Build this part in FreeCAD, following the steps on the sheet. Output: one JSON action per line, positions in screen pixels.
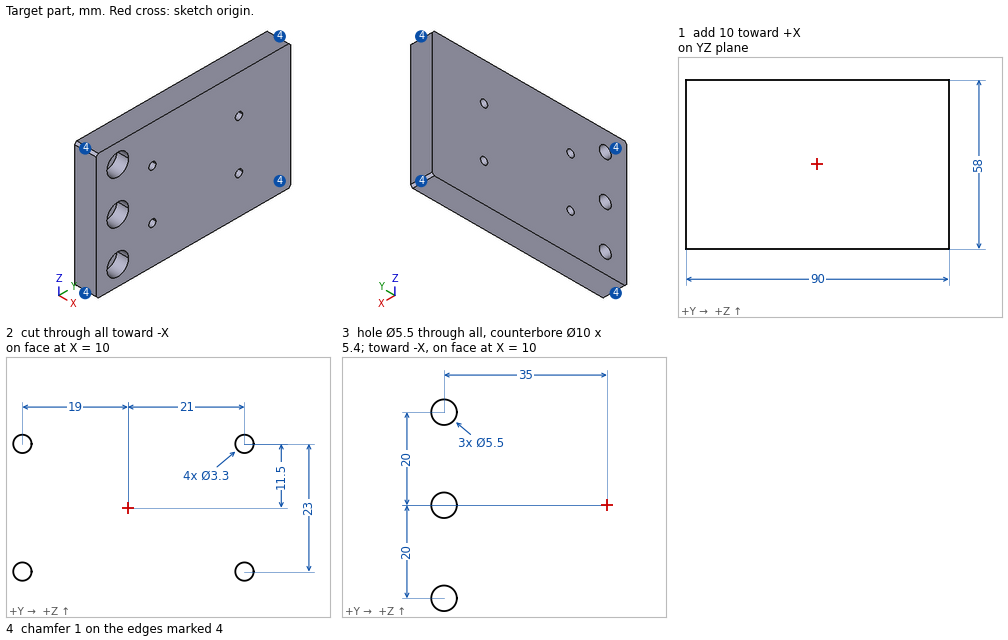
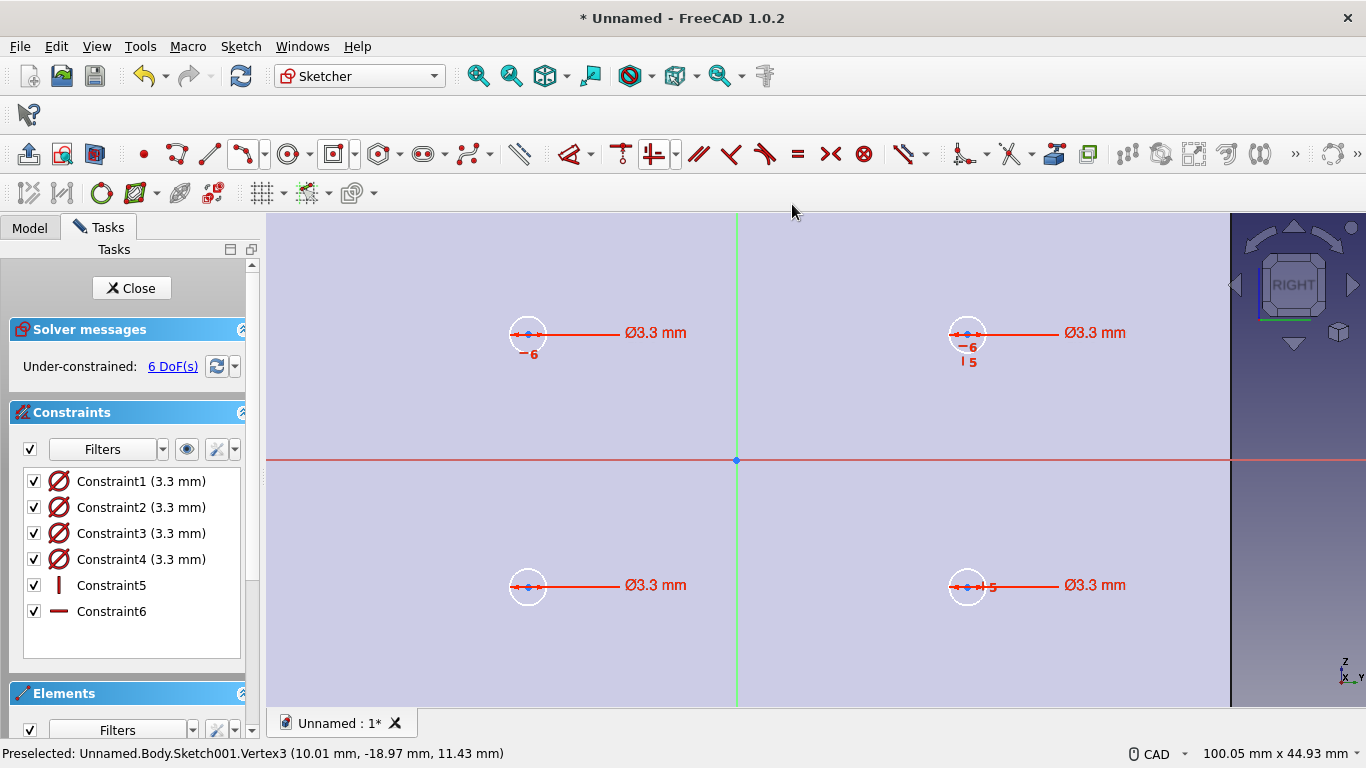
{"action": "left_click", "coordinate": [528, 335]}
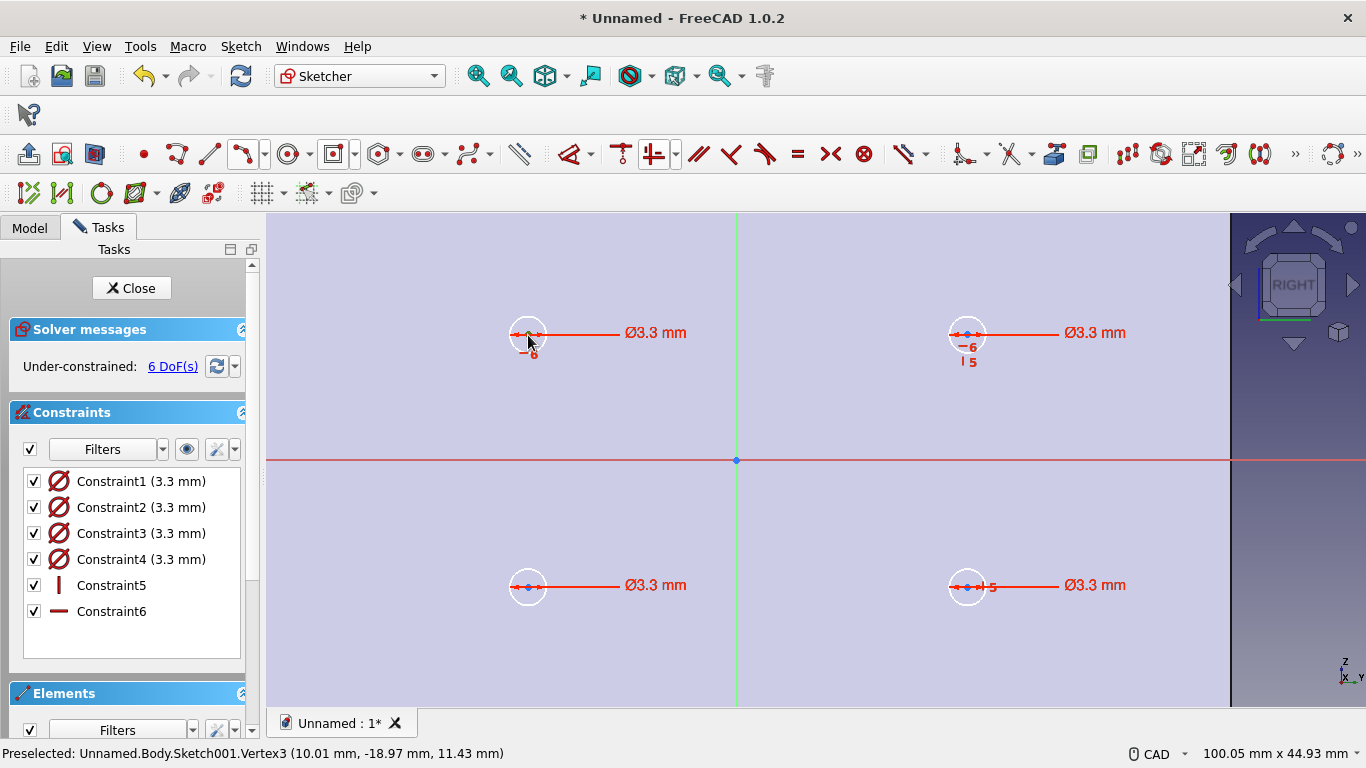
{"action": "left_click", "coordinate": [528, 587]}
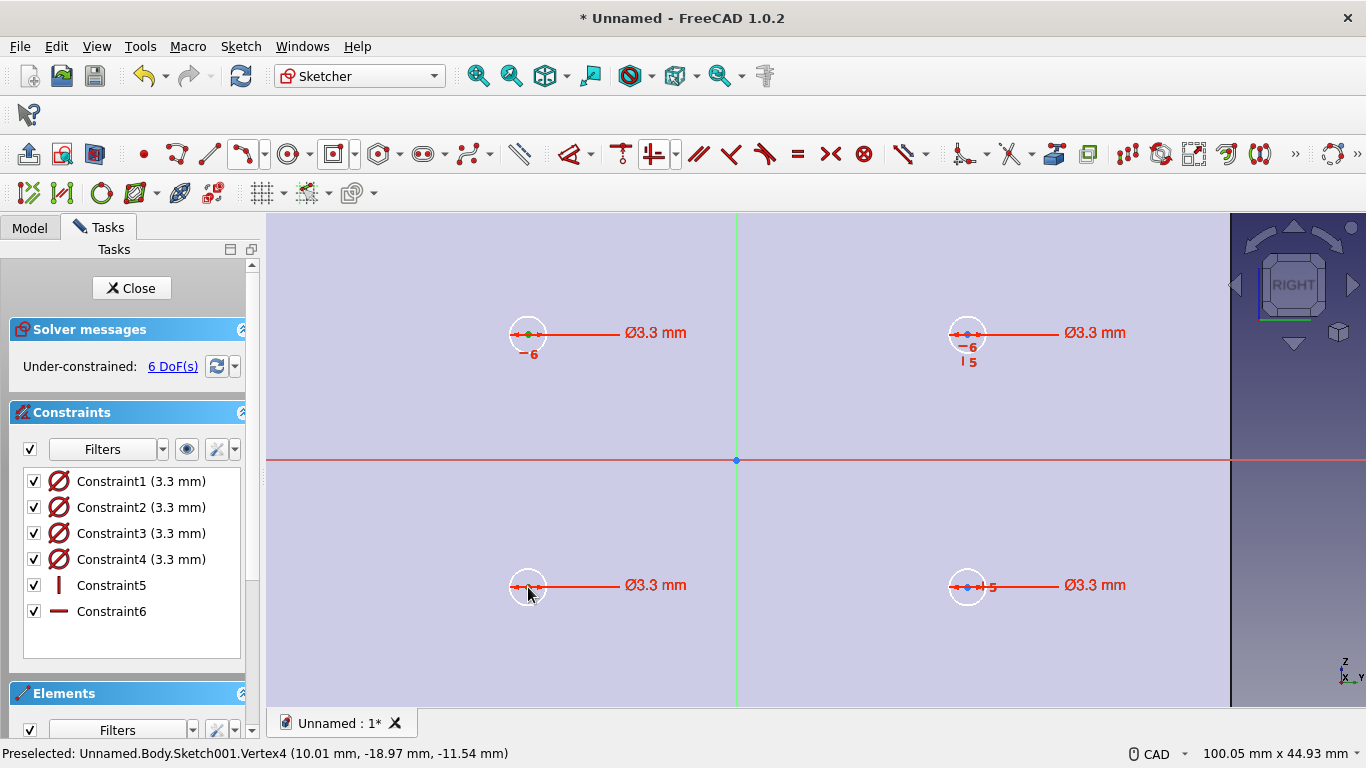
{"action": "left_click", "coordinate": [676, 154]}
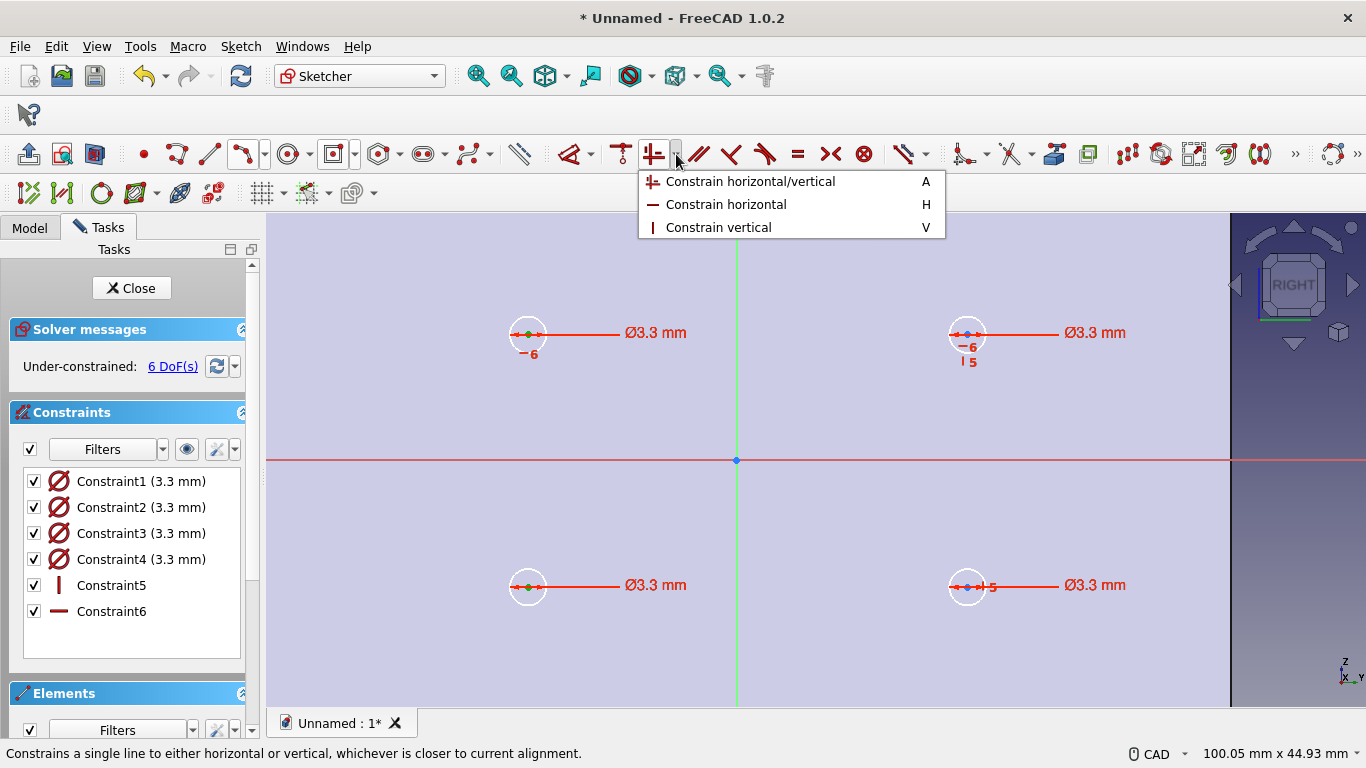
{"action": "left_click", "coordinate": [792, 228]}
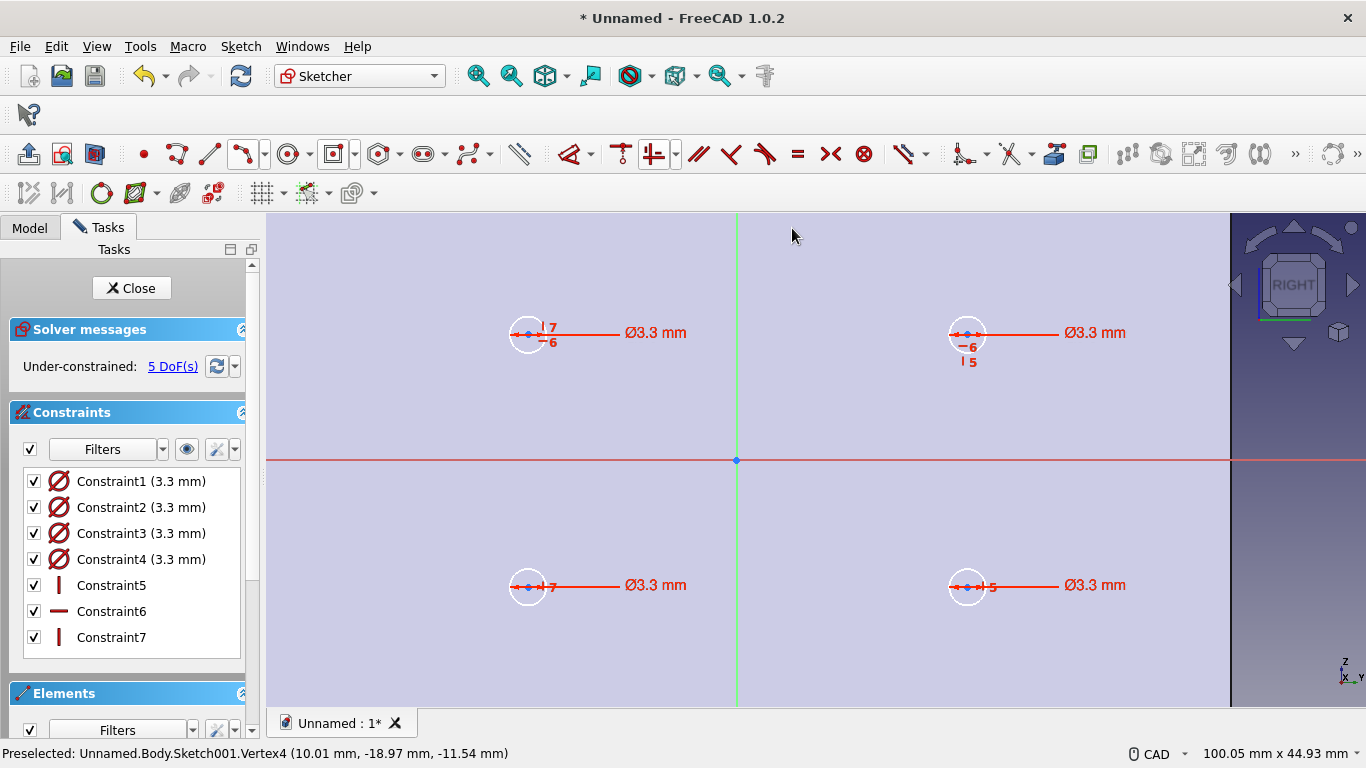
{"action": "left_click", "coordinate": [968, 587]}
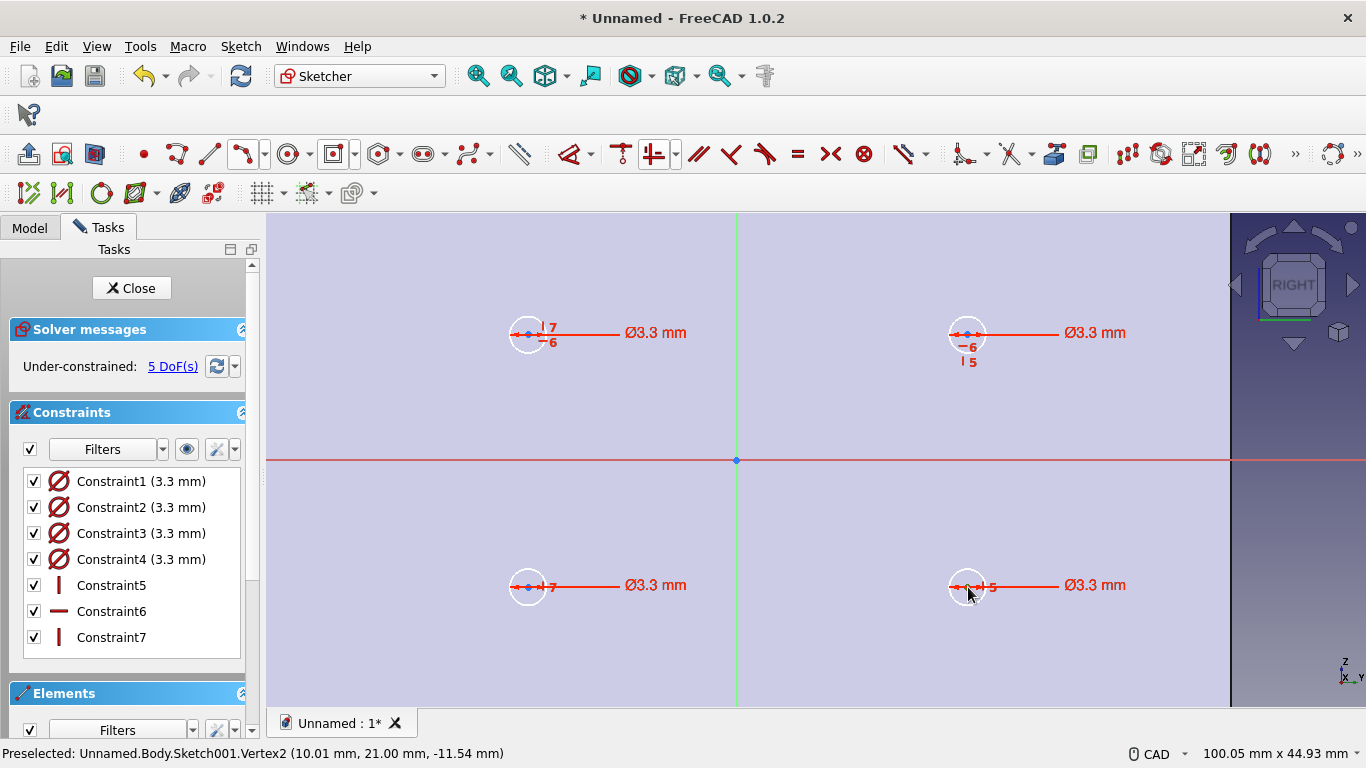
{"action": "left_click", "coordinate": [528, 587]}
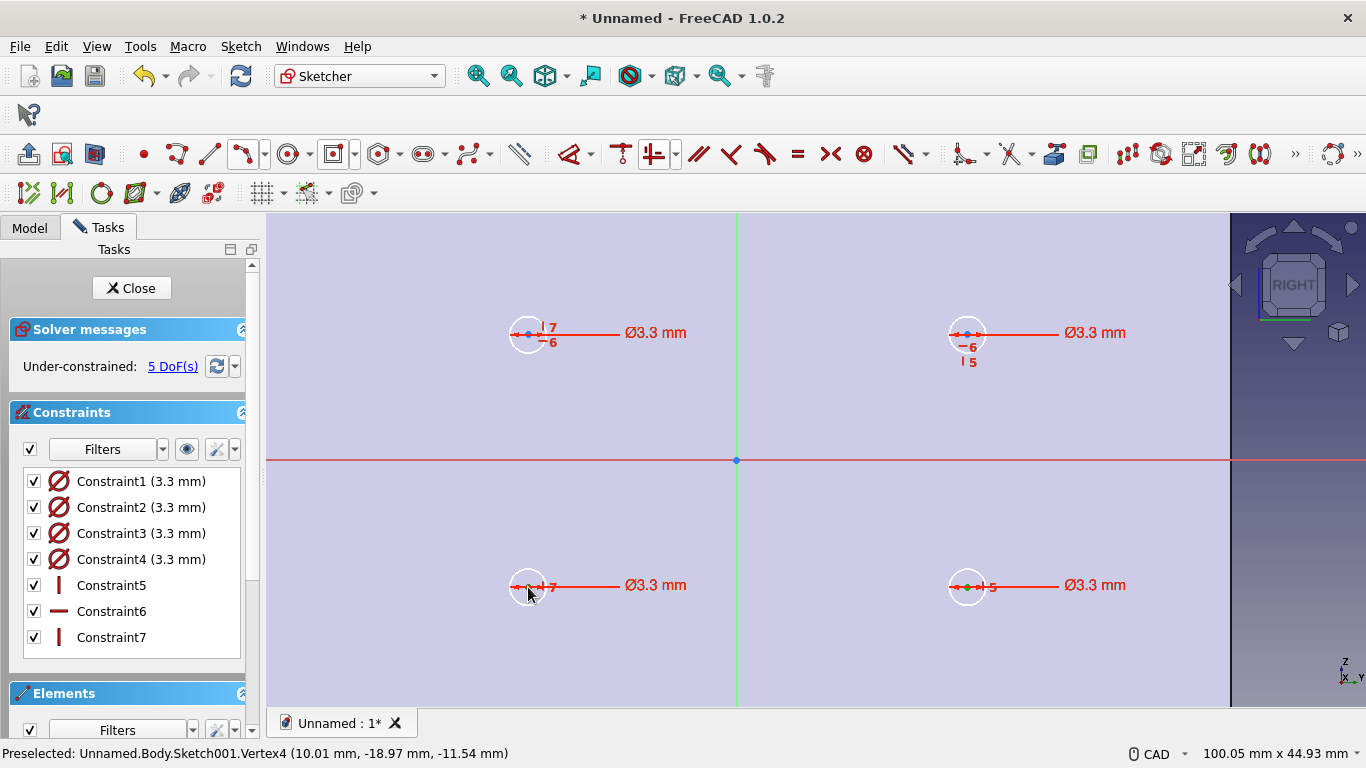
{"action": "left_click", "coordinate": [676, 154]}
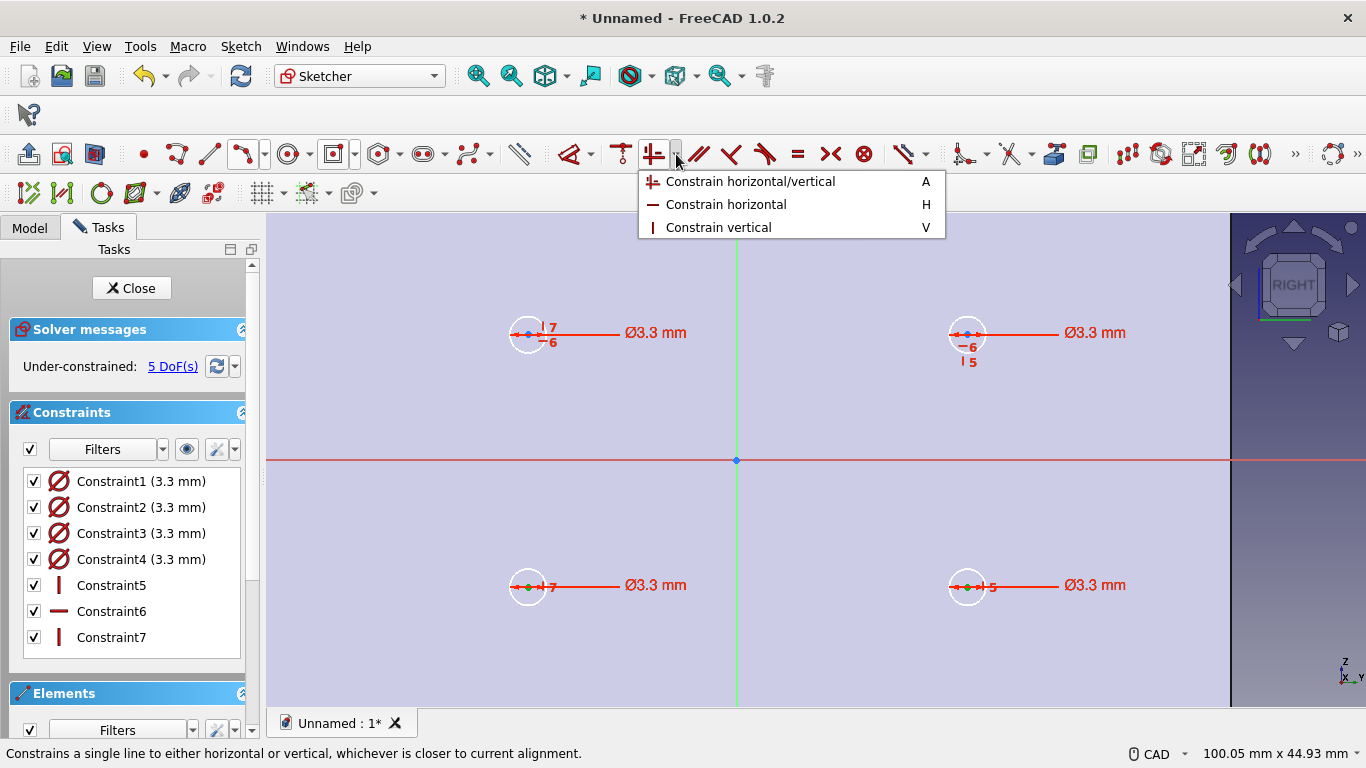
{"action": "left_click", "coordinate": [792, 204]}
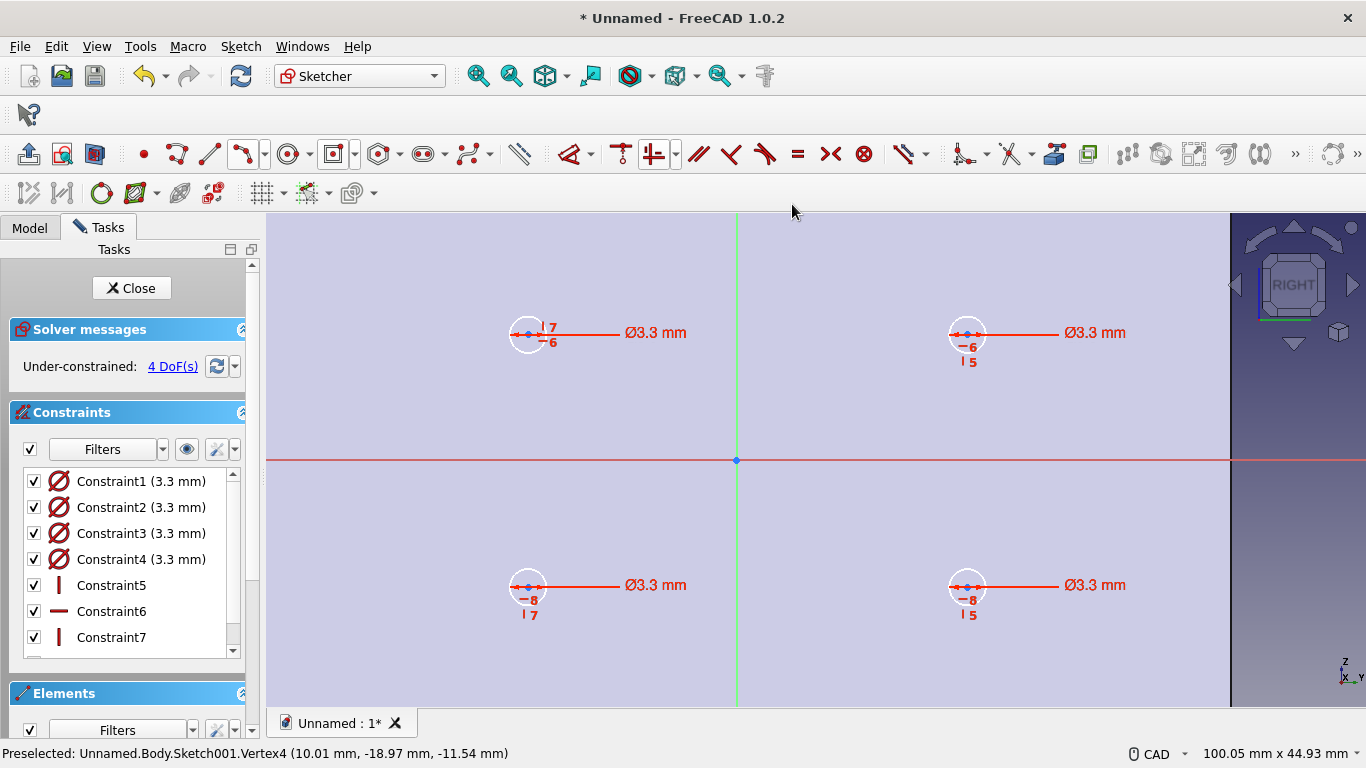
{"action": "left_click", "coordinate": [968, 335]}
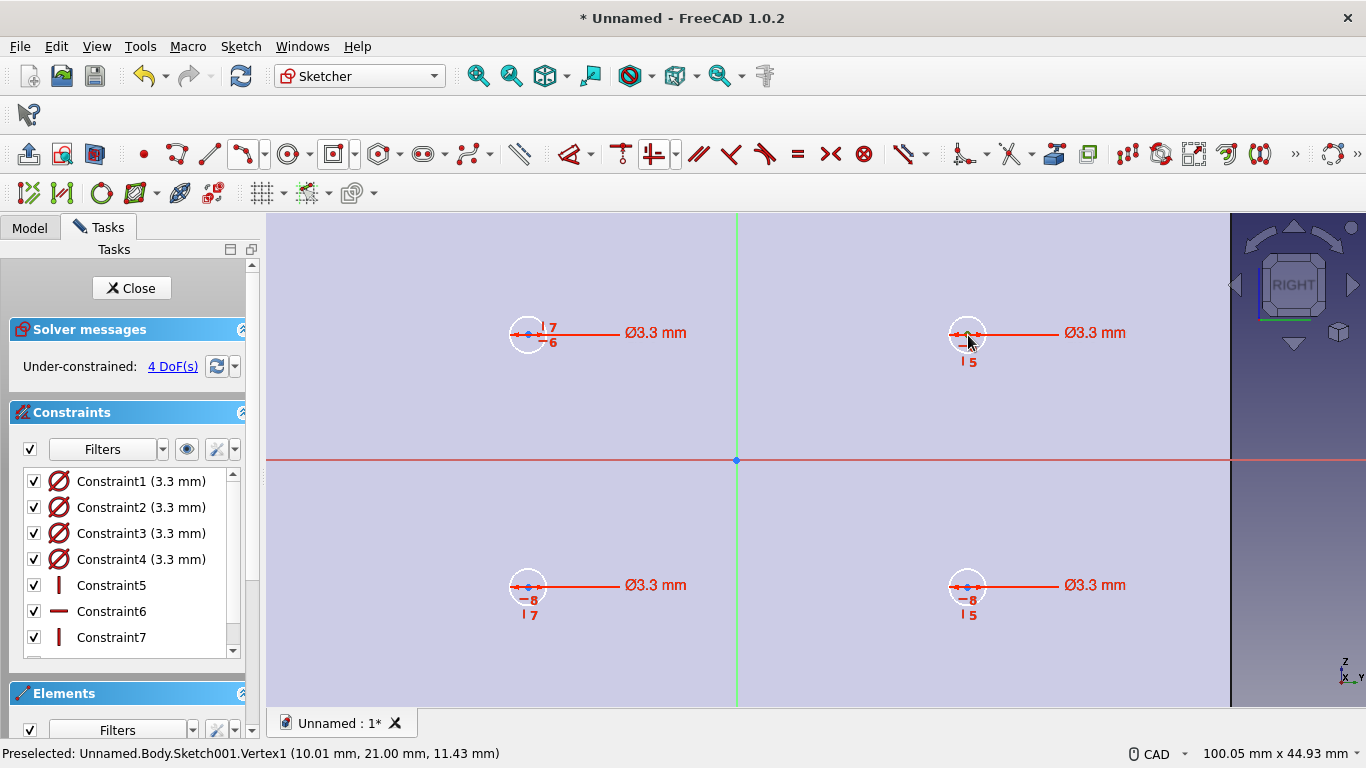
{"action": "key", "text": "l"}